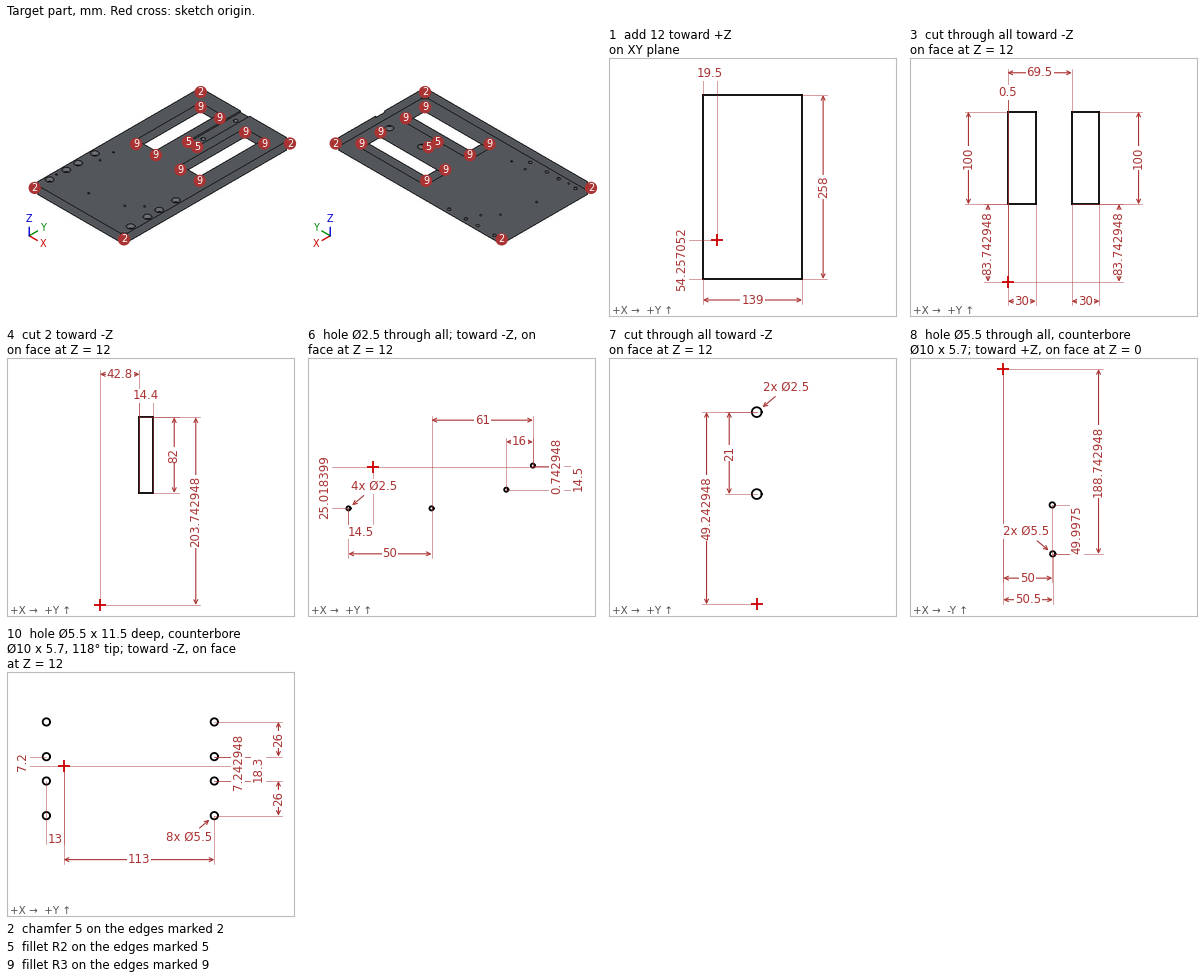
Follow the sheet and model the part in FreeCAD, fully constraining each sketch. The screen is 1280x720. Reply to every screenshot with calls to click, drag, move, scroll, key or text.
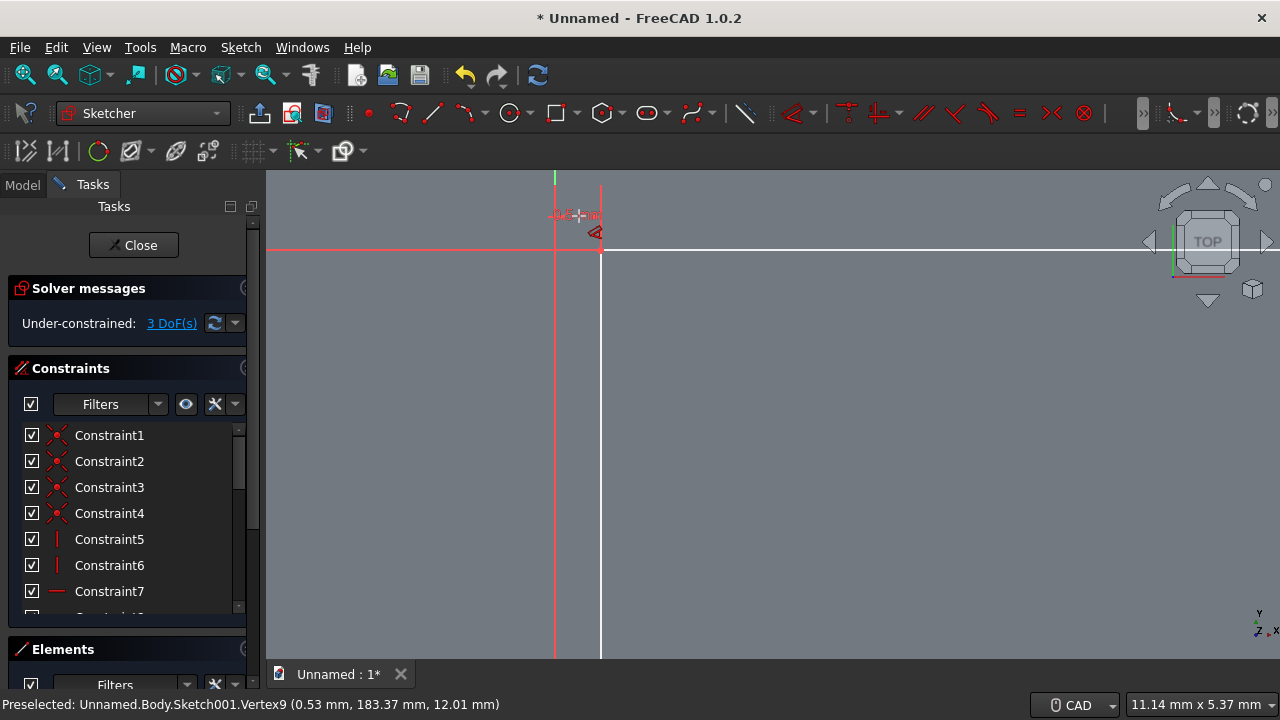
scroll(704, 414, down, 15)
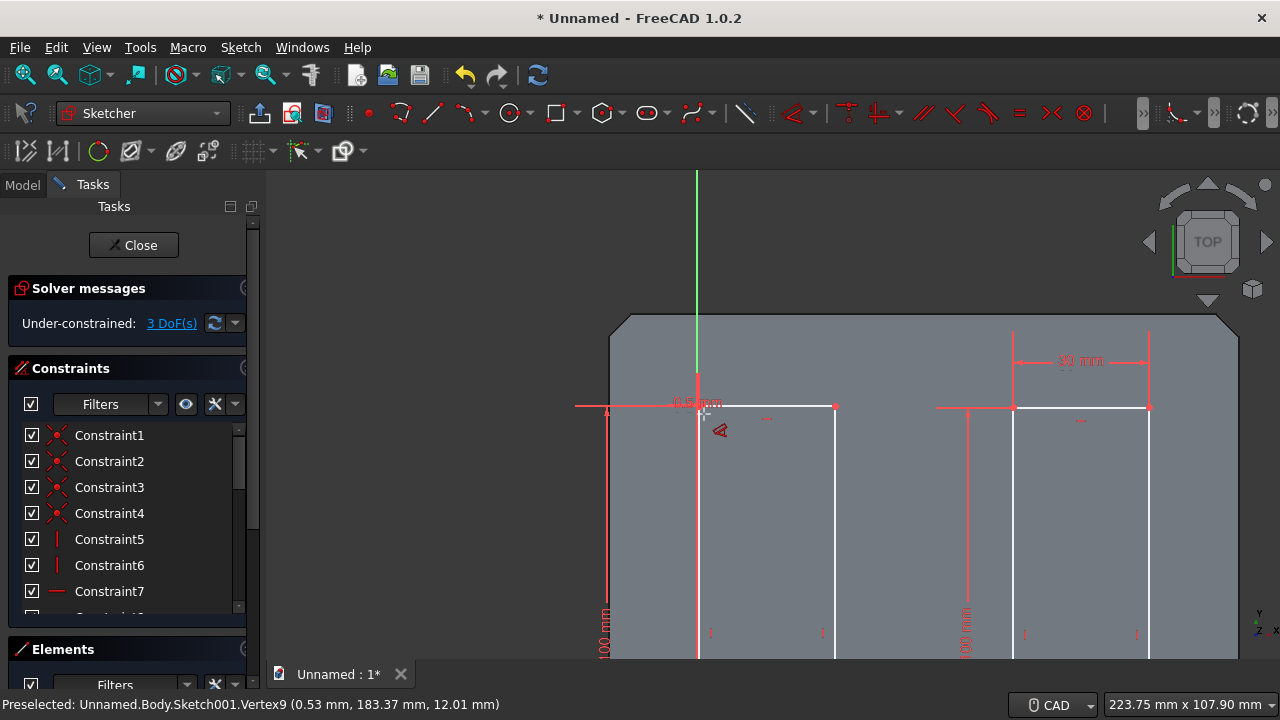
scroll(578, 198, down, 5)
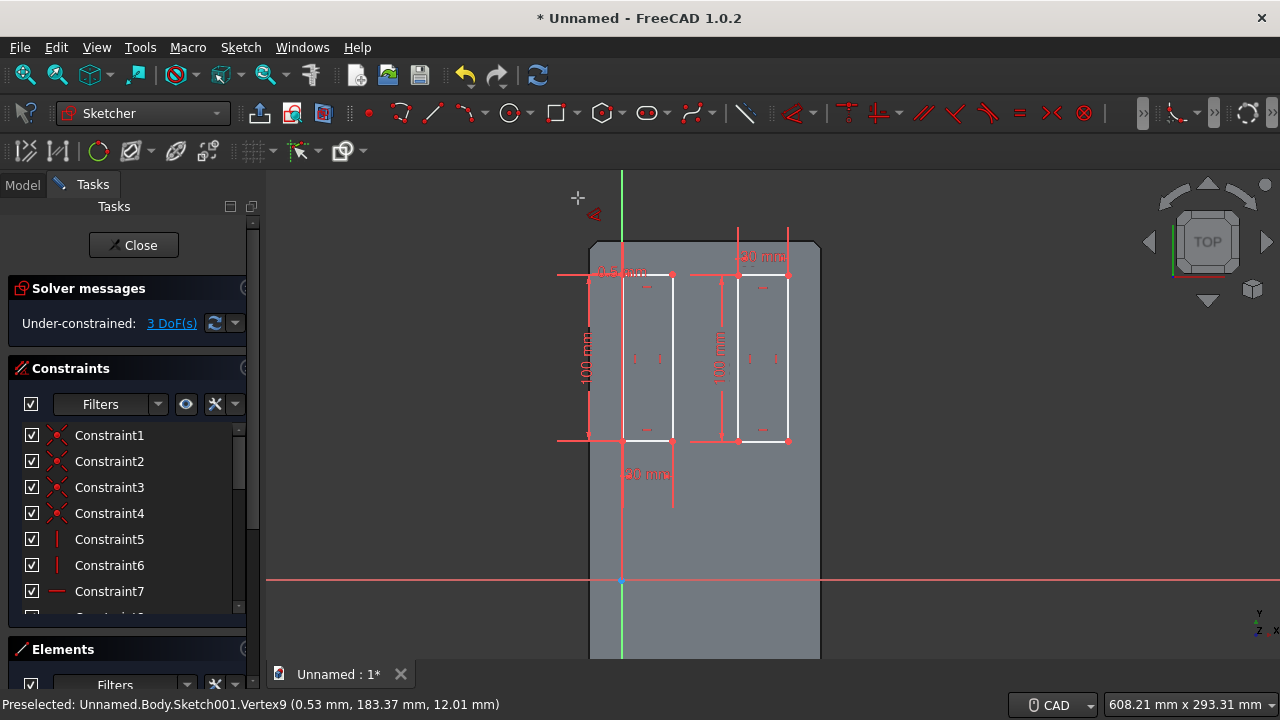
click(738, 275)
click(680, 614)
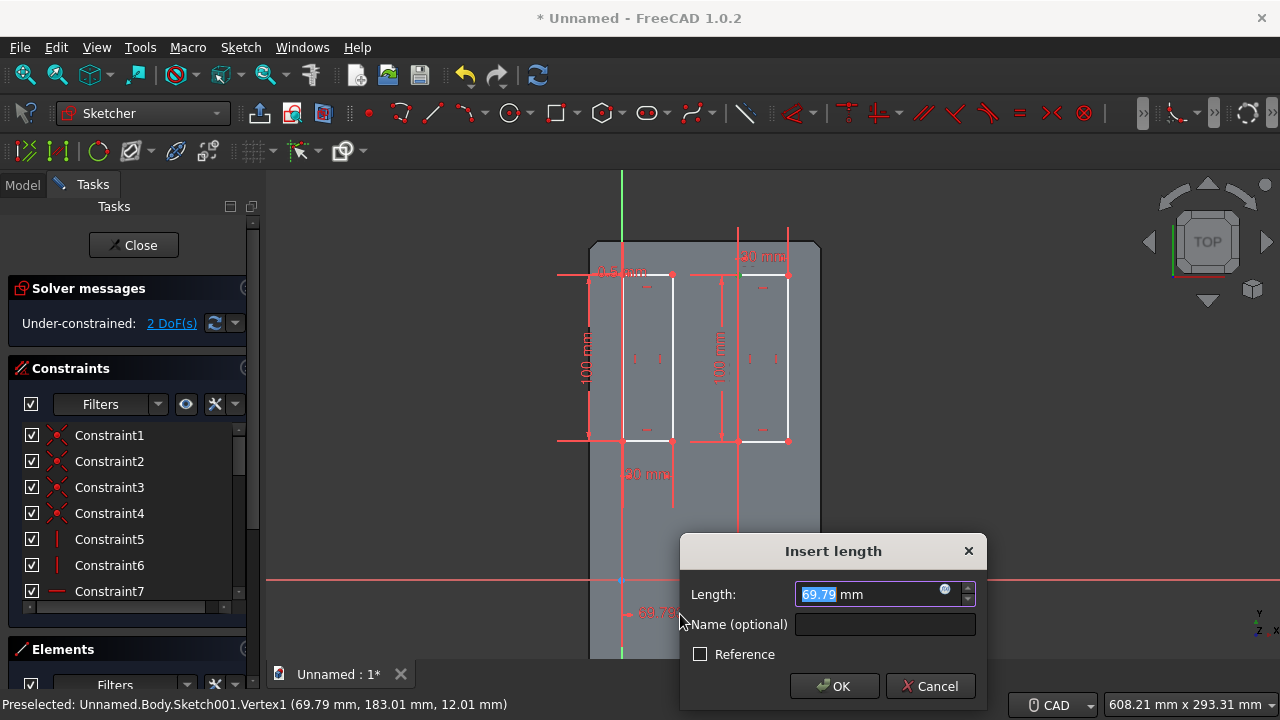
text(69.5)
key(Return)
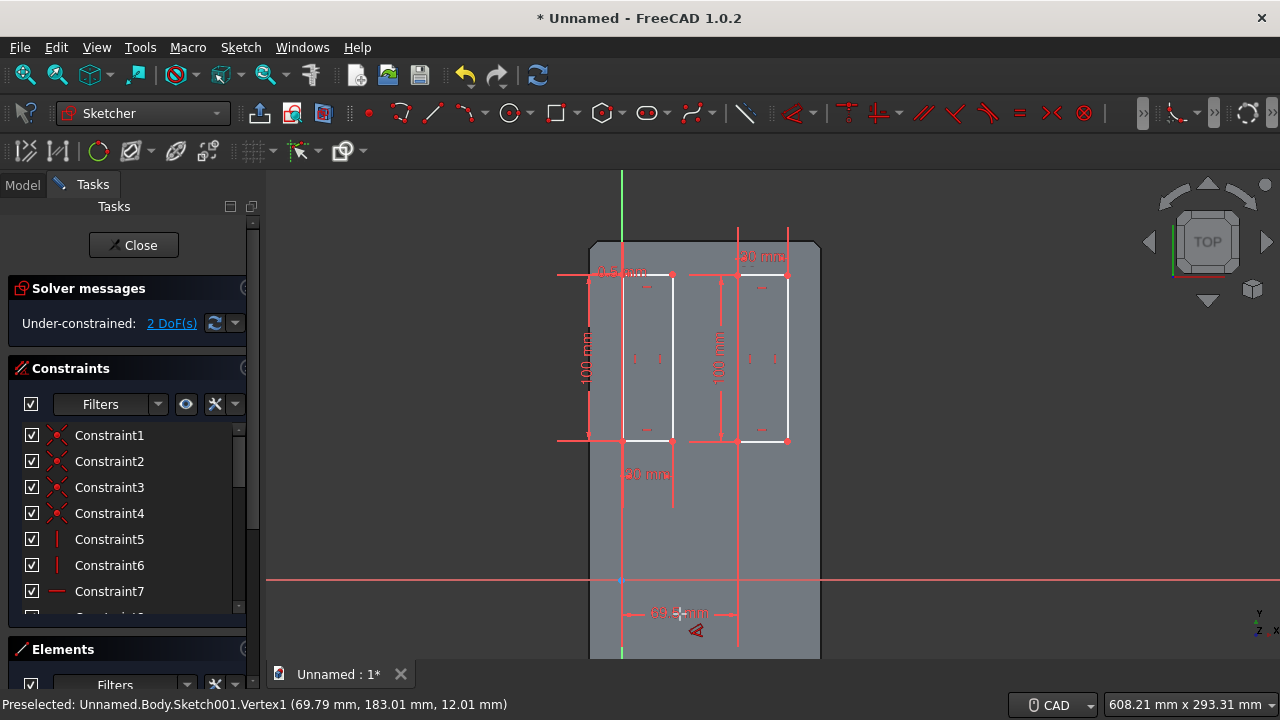
click(738, 442)
click(588, 511)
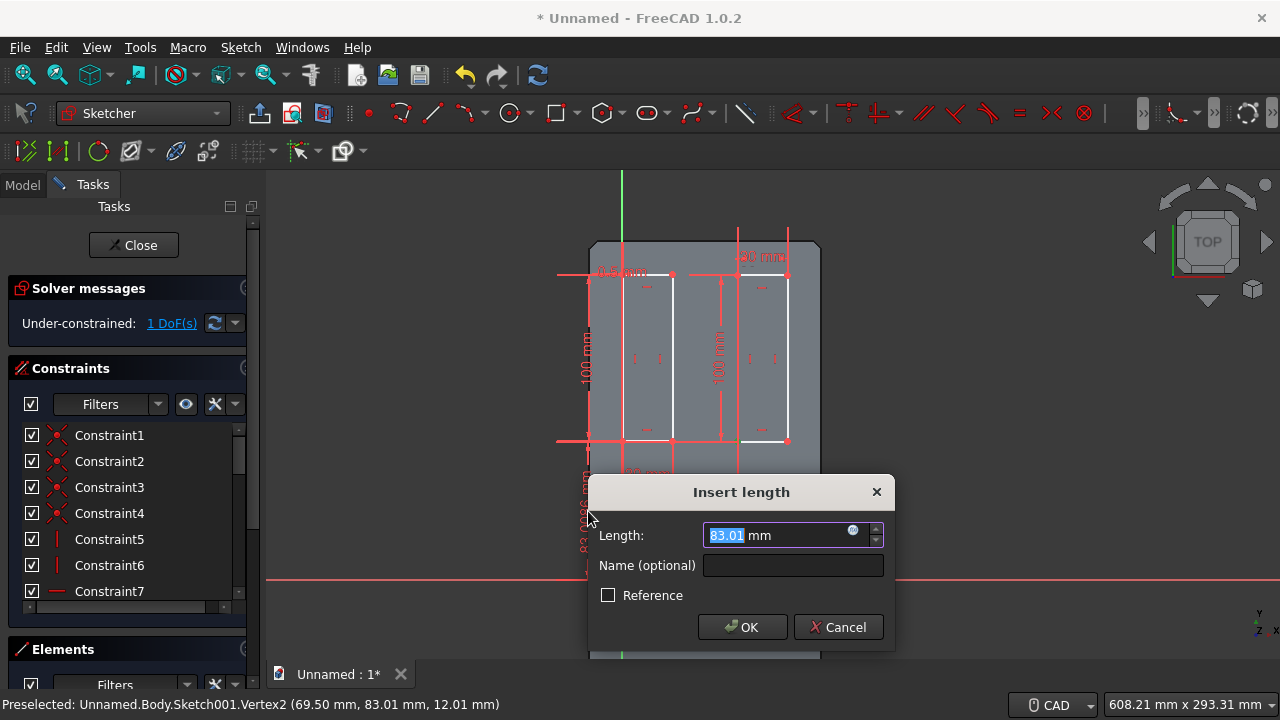
text(83.742948)
key(Return)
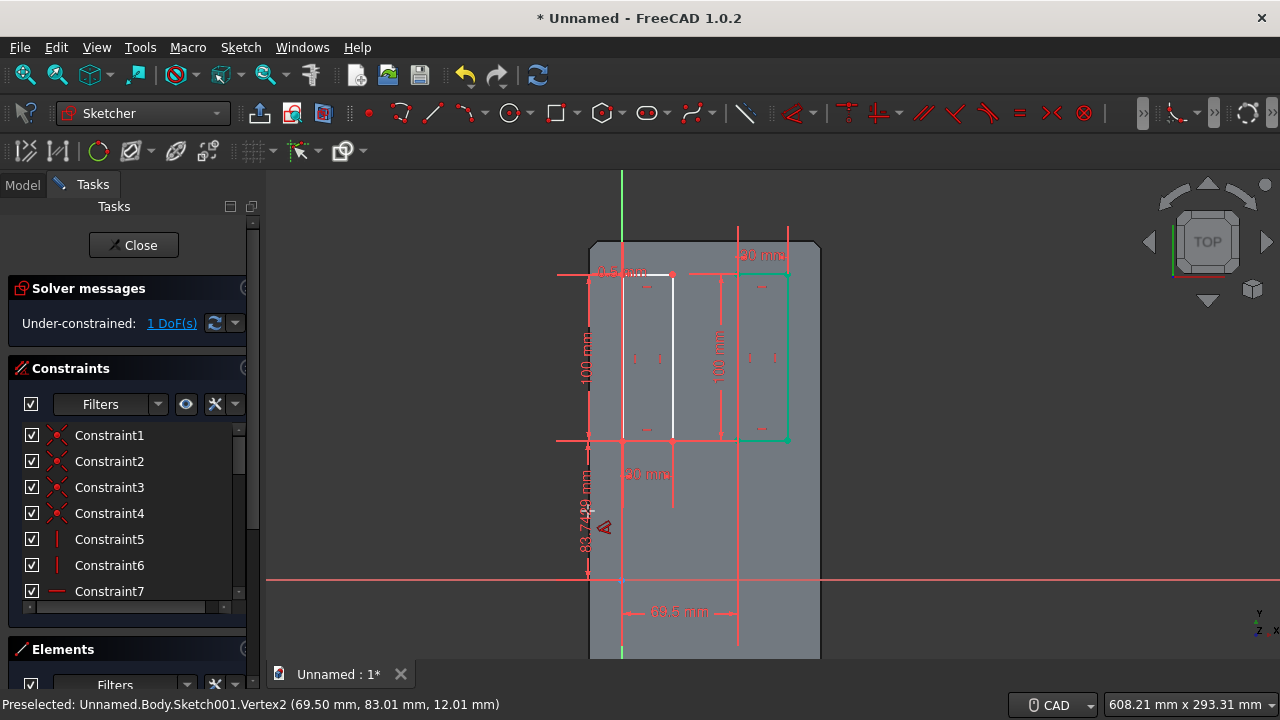
click(623, 441)
click(588, 543)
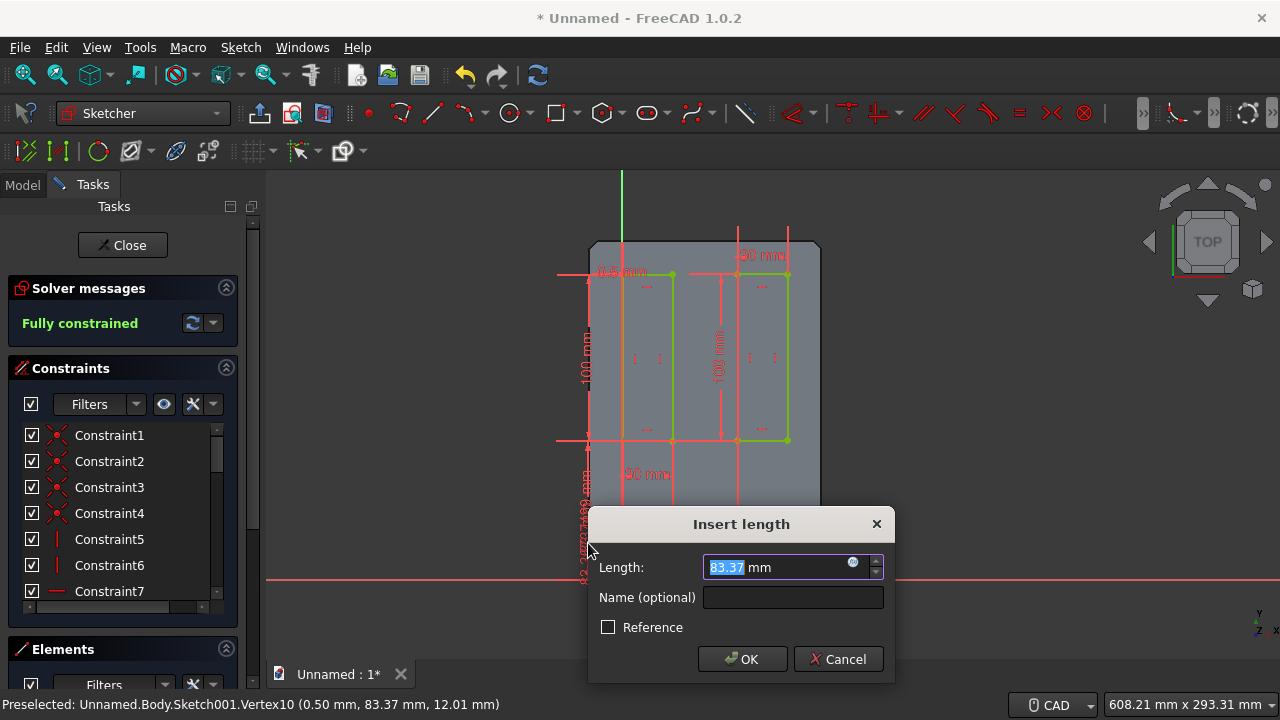
text(83.742948)
key(Return)
key(Escape)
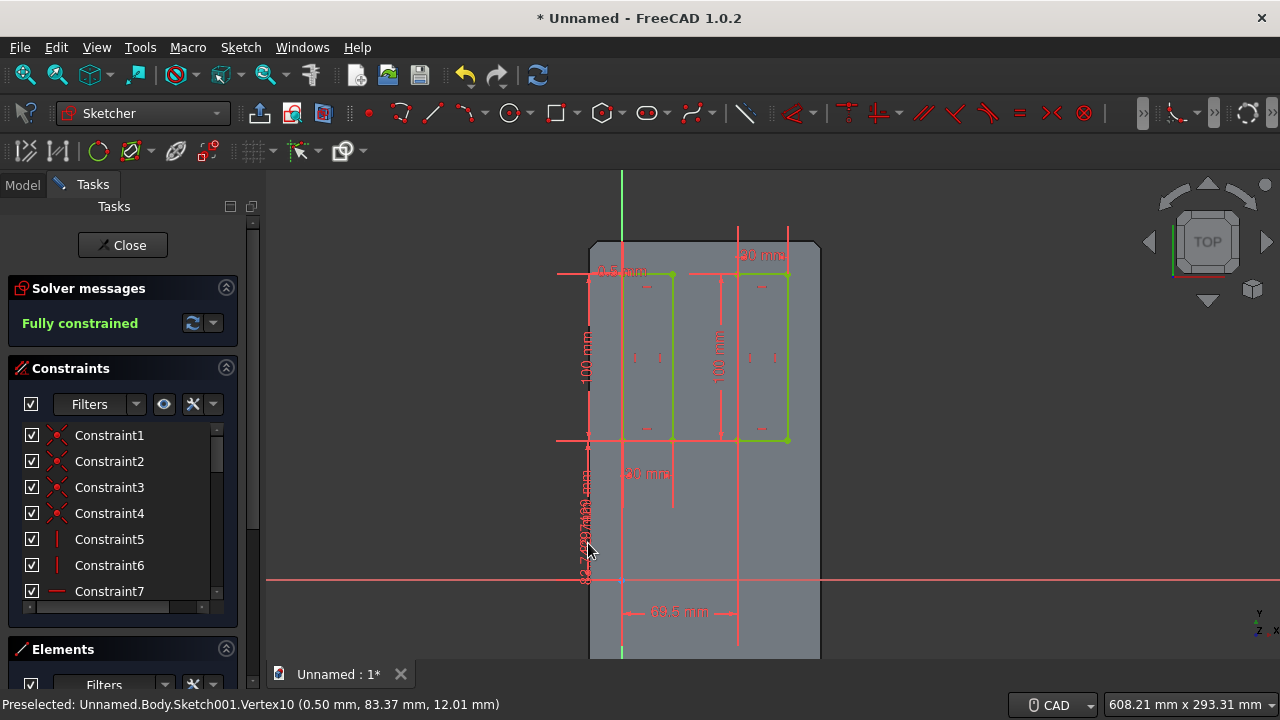
click(123, 245)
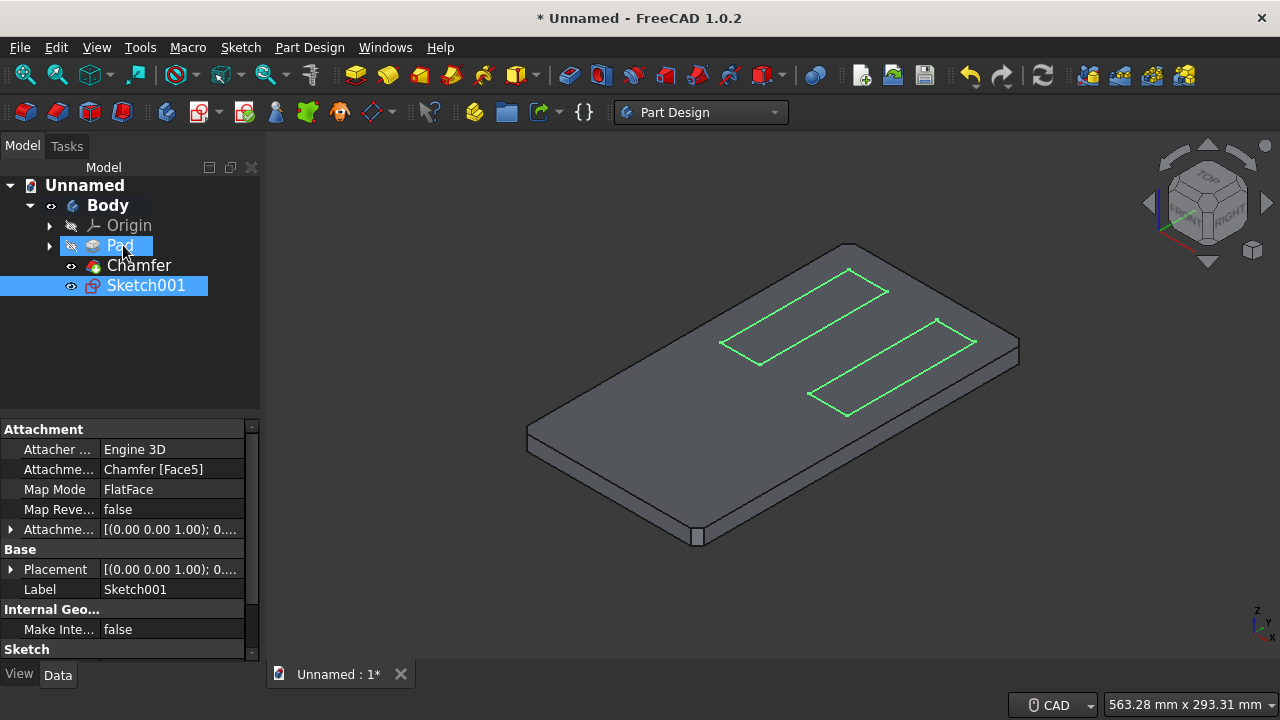
click(570, 76)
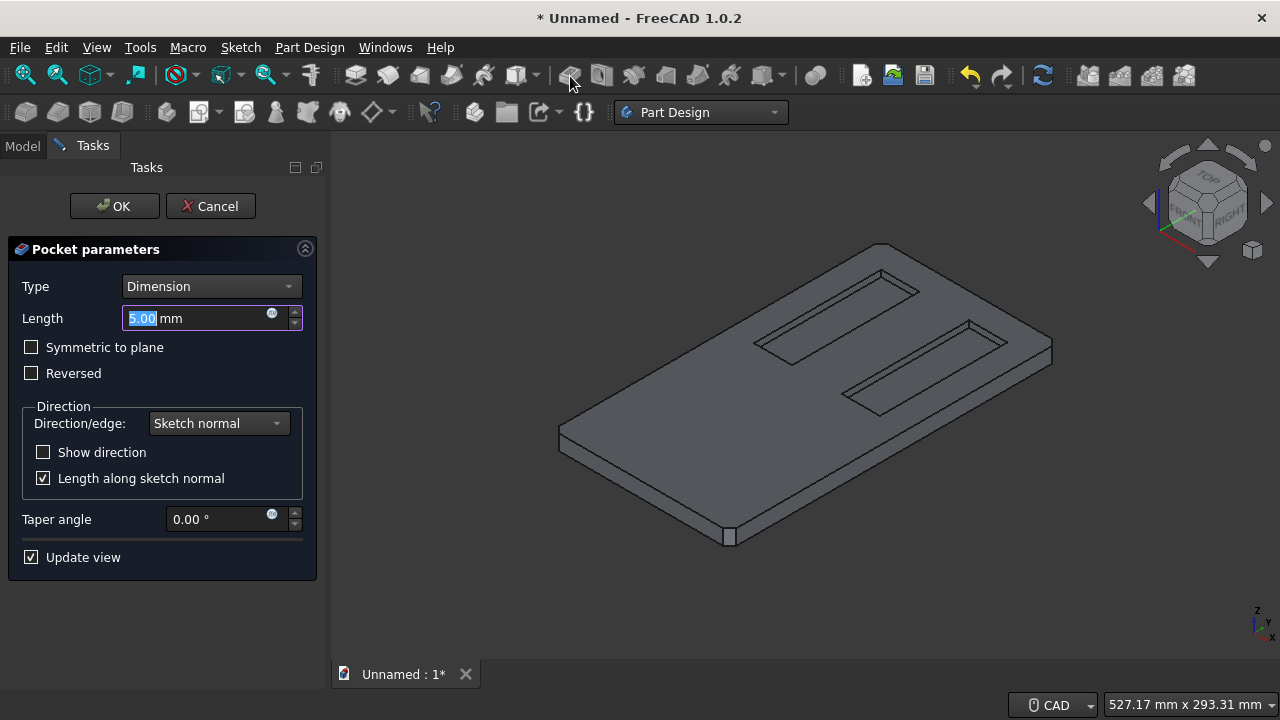
click(212, 286)